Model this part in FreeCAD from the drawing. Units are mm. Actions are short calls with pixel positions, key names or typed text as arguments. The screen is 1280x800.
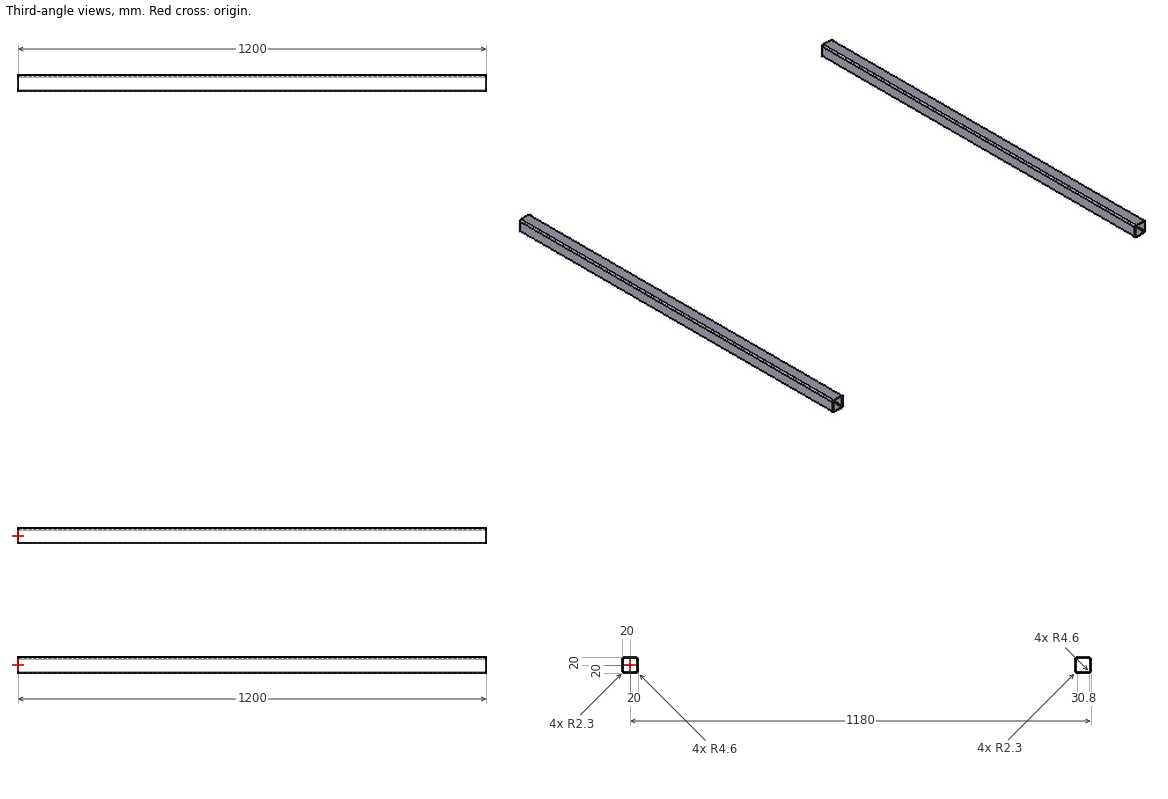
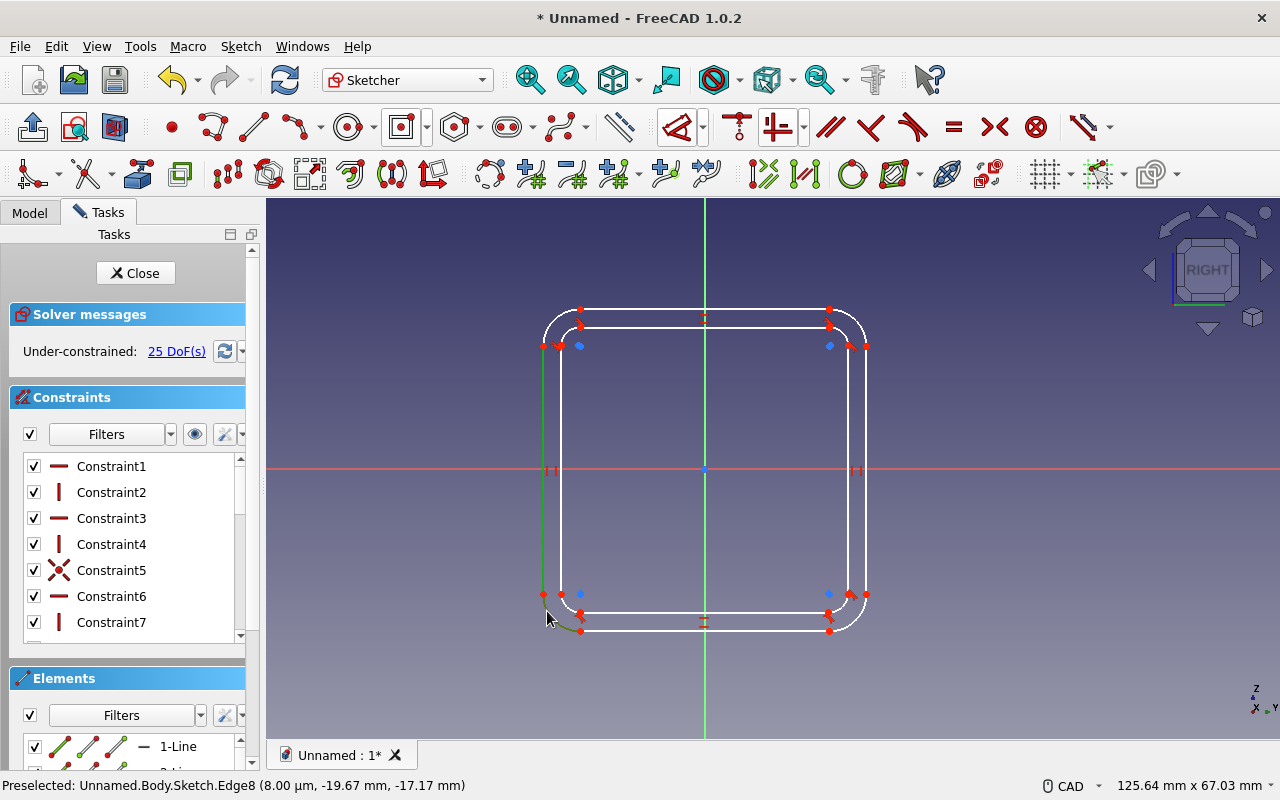
key(t)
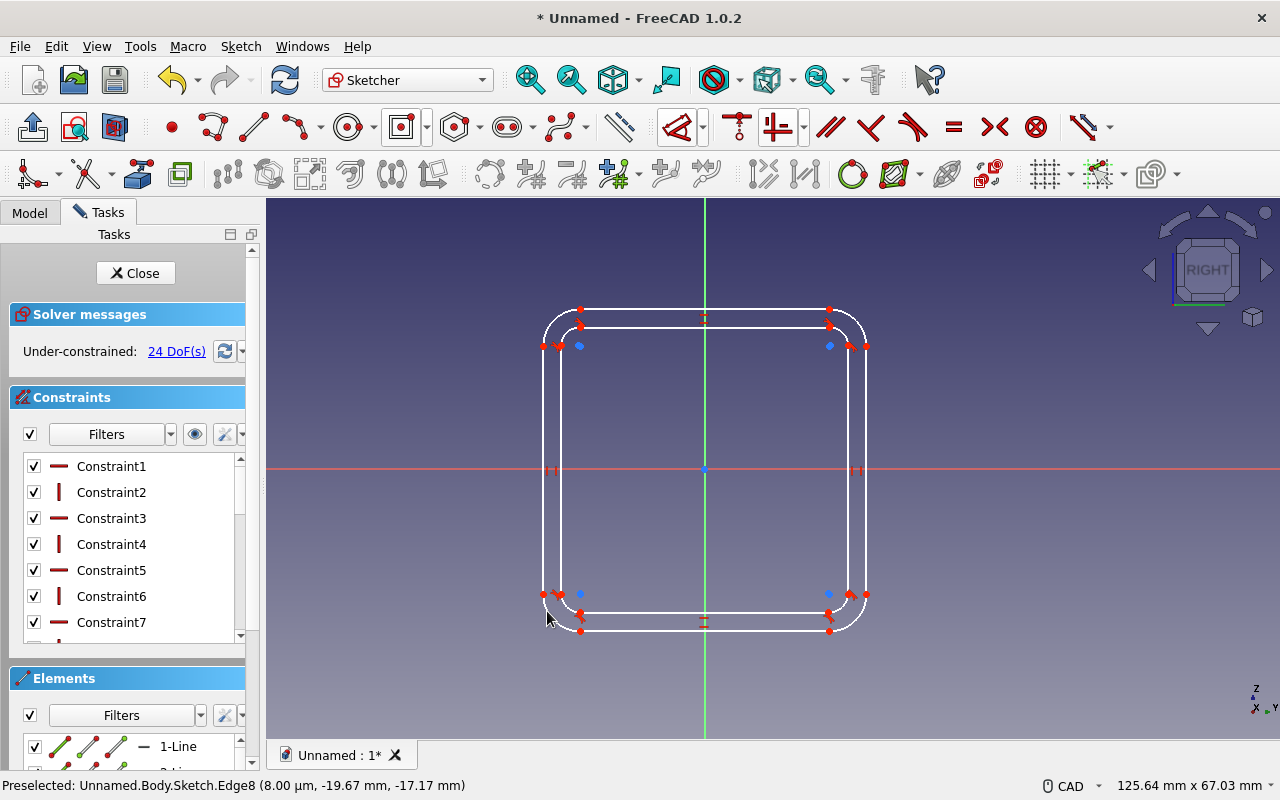
click(754, 613)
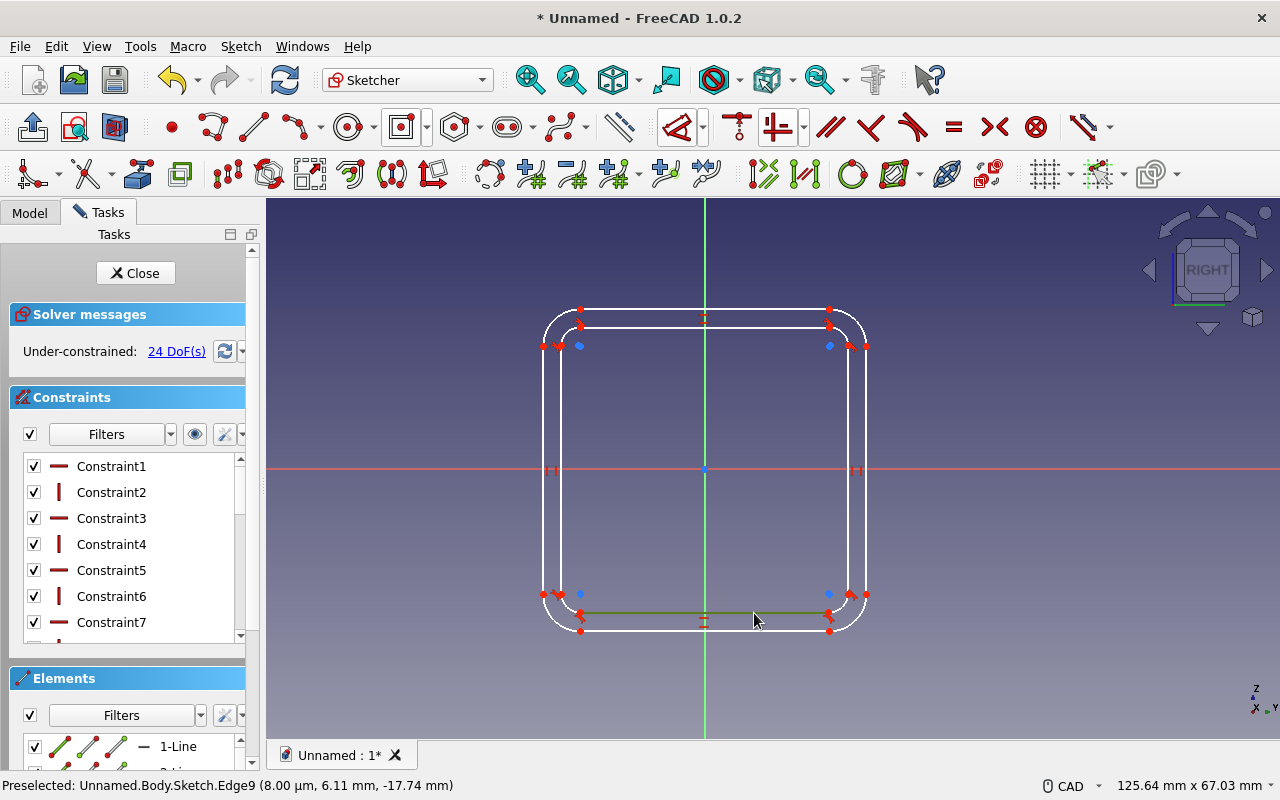
click(567, 607)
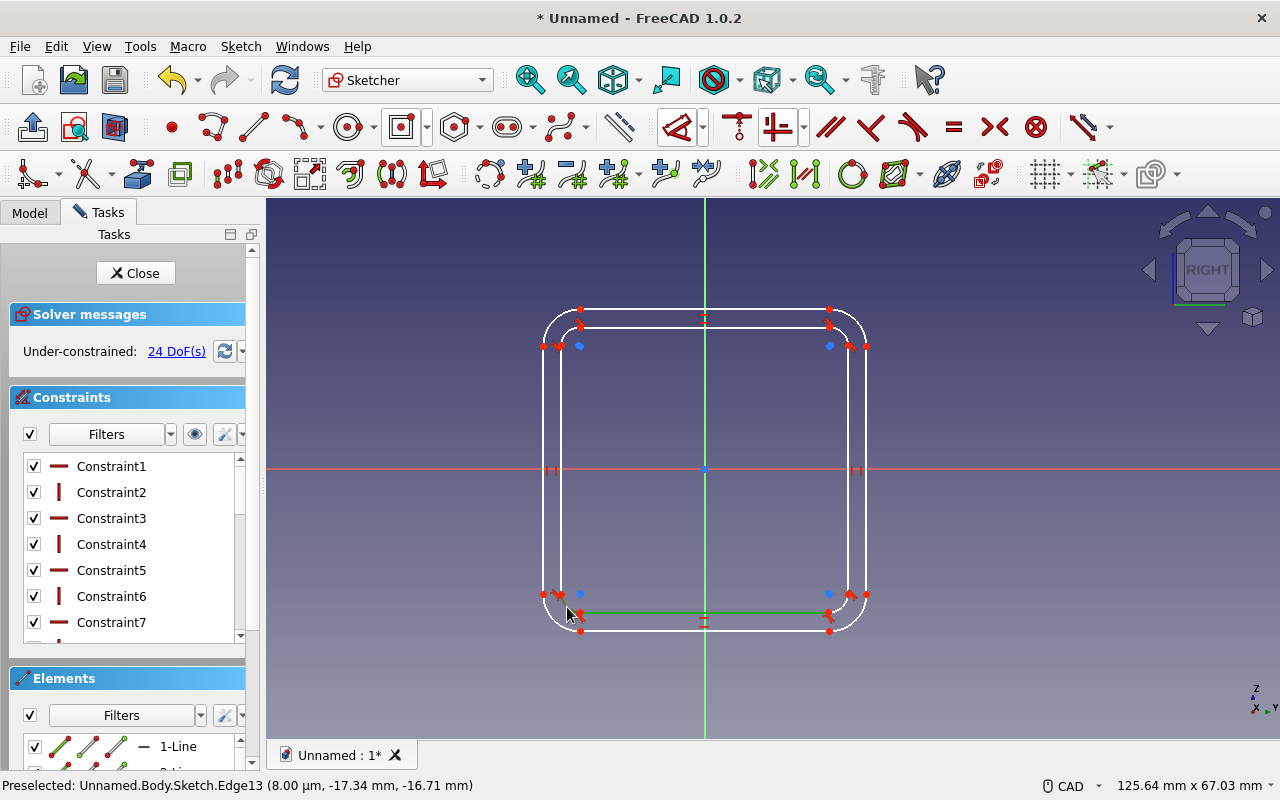
key(t)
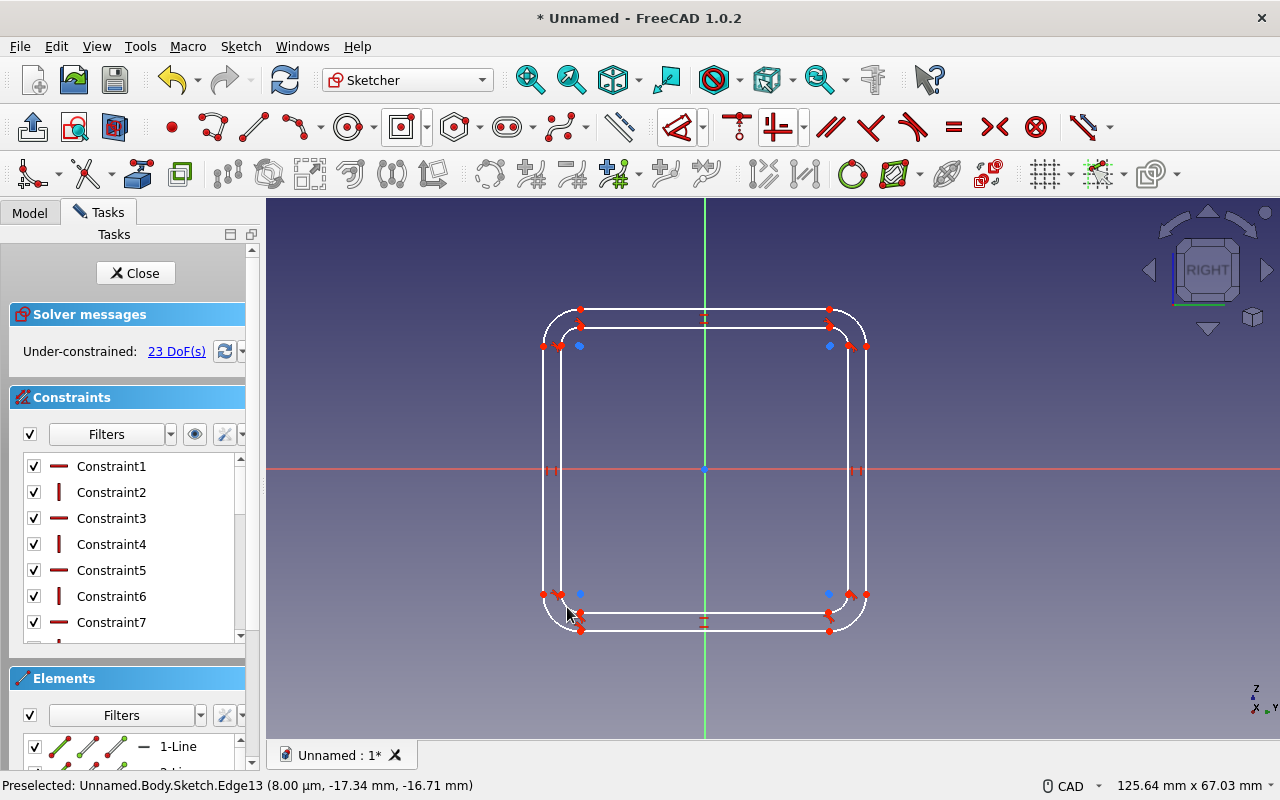
click(754, 613)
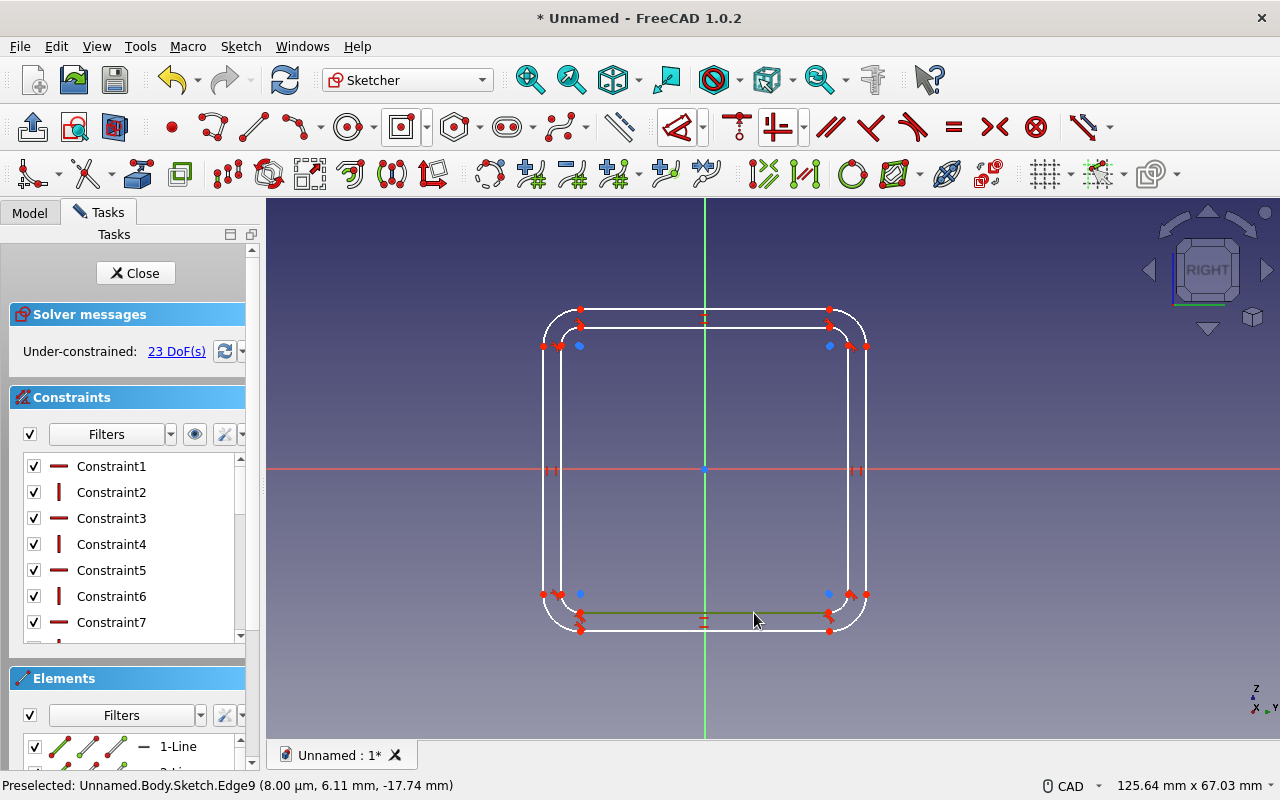
click(842, 607)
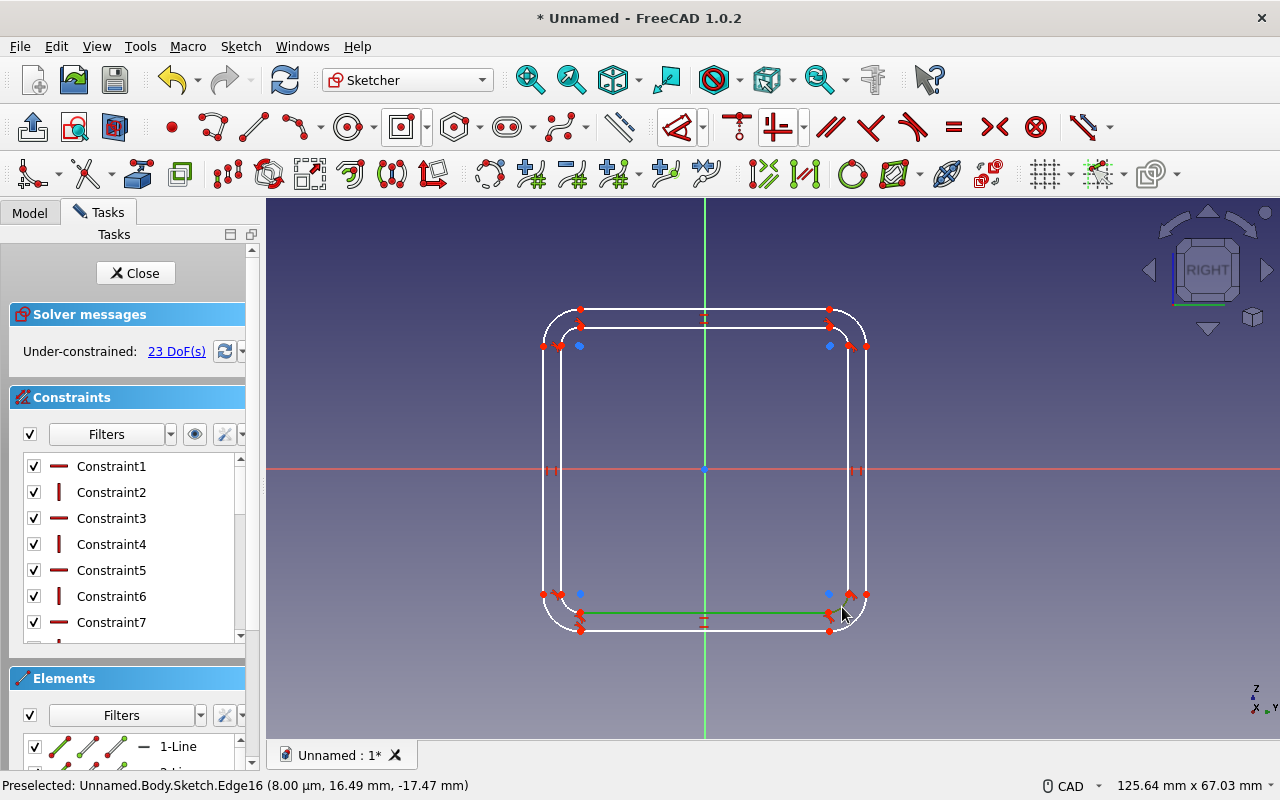
click(913, 128)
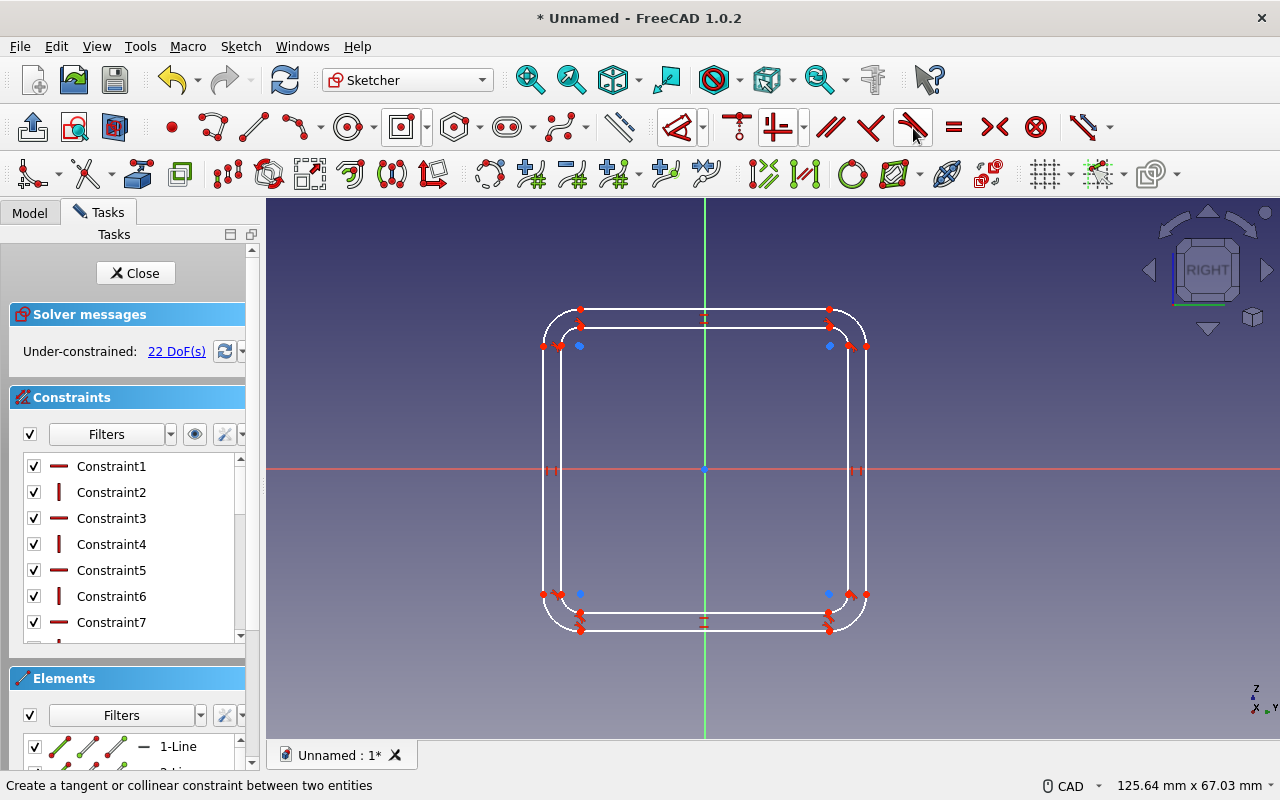
click(561, 520)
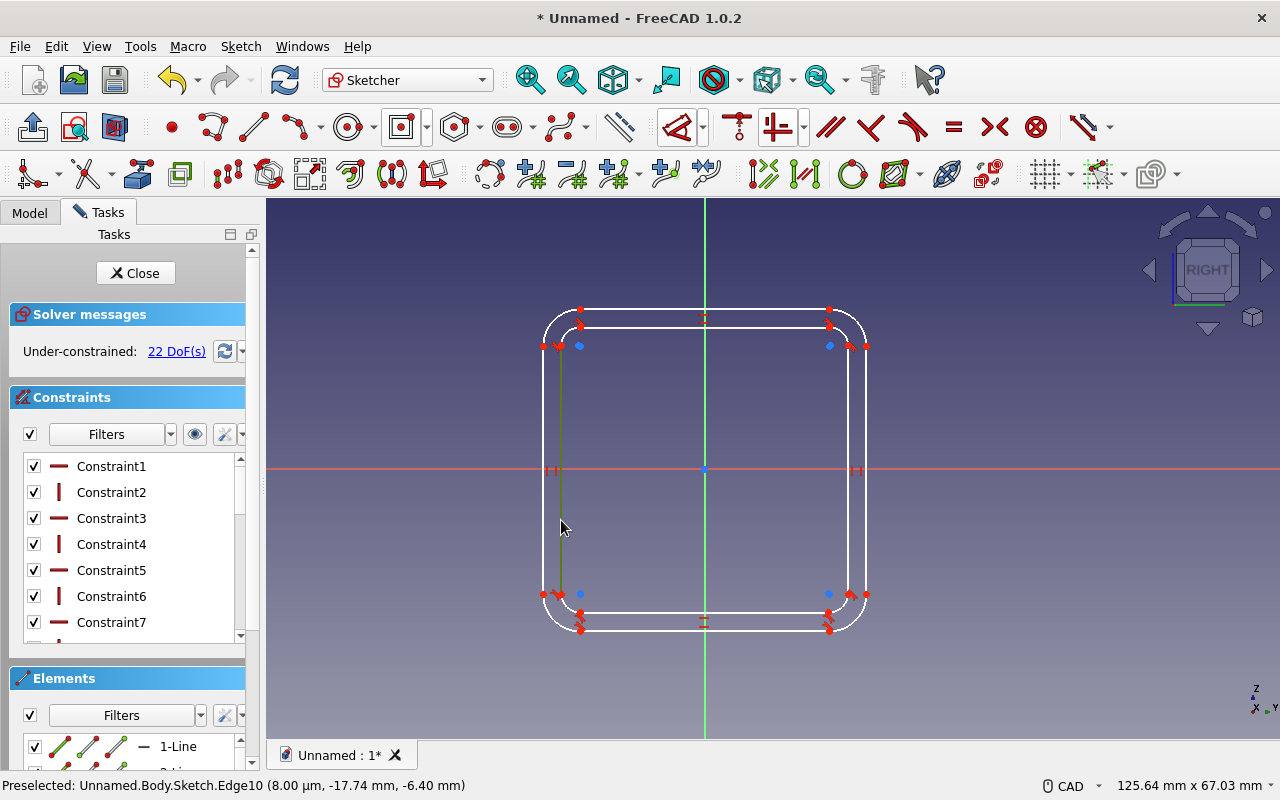
click(567, 607)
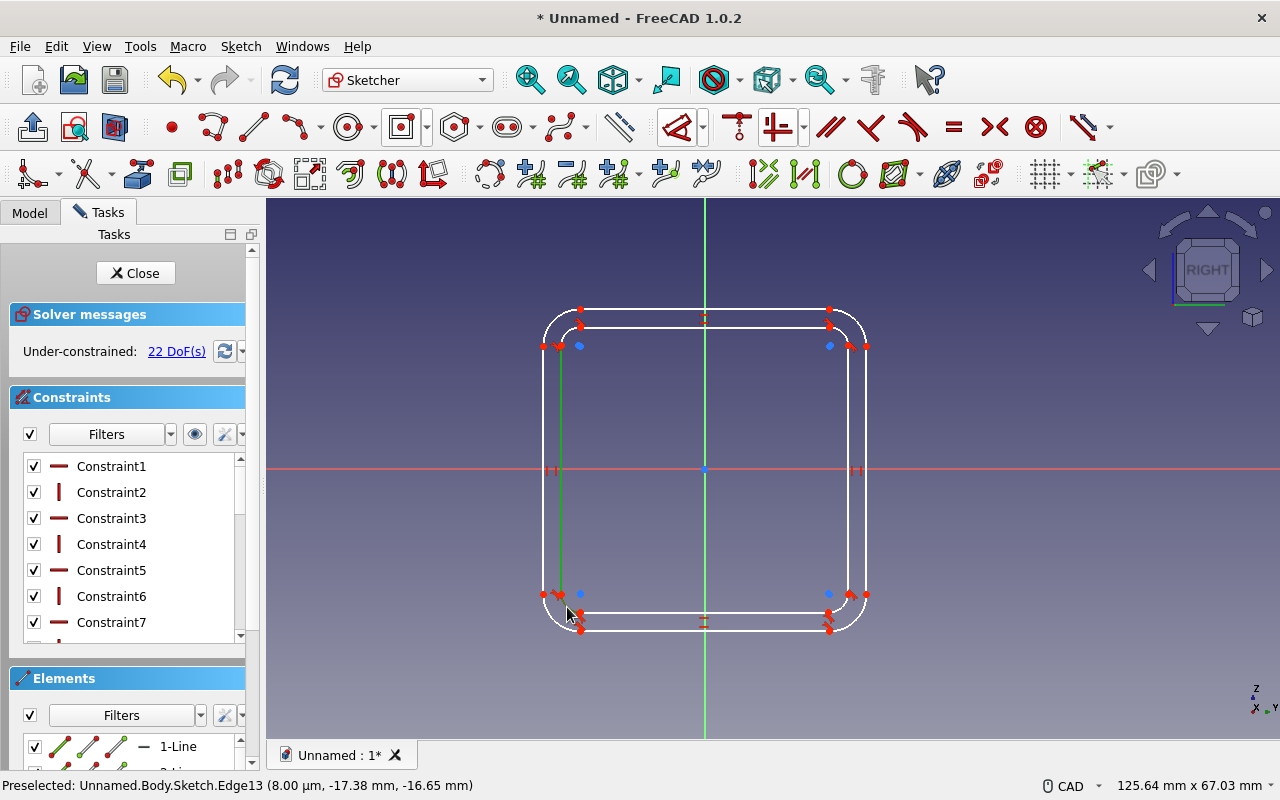
click(913, 128)